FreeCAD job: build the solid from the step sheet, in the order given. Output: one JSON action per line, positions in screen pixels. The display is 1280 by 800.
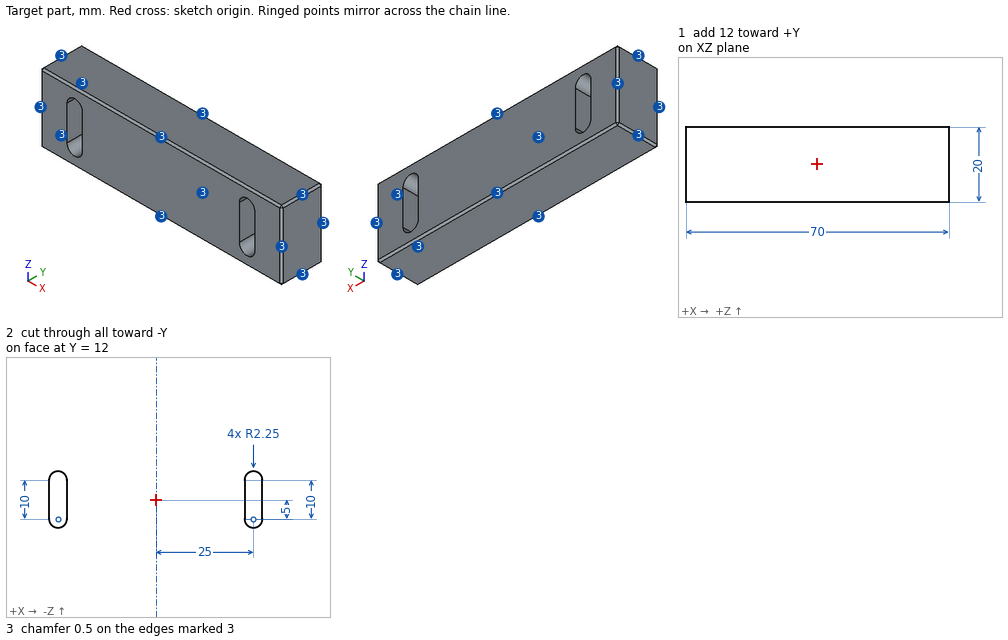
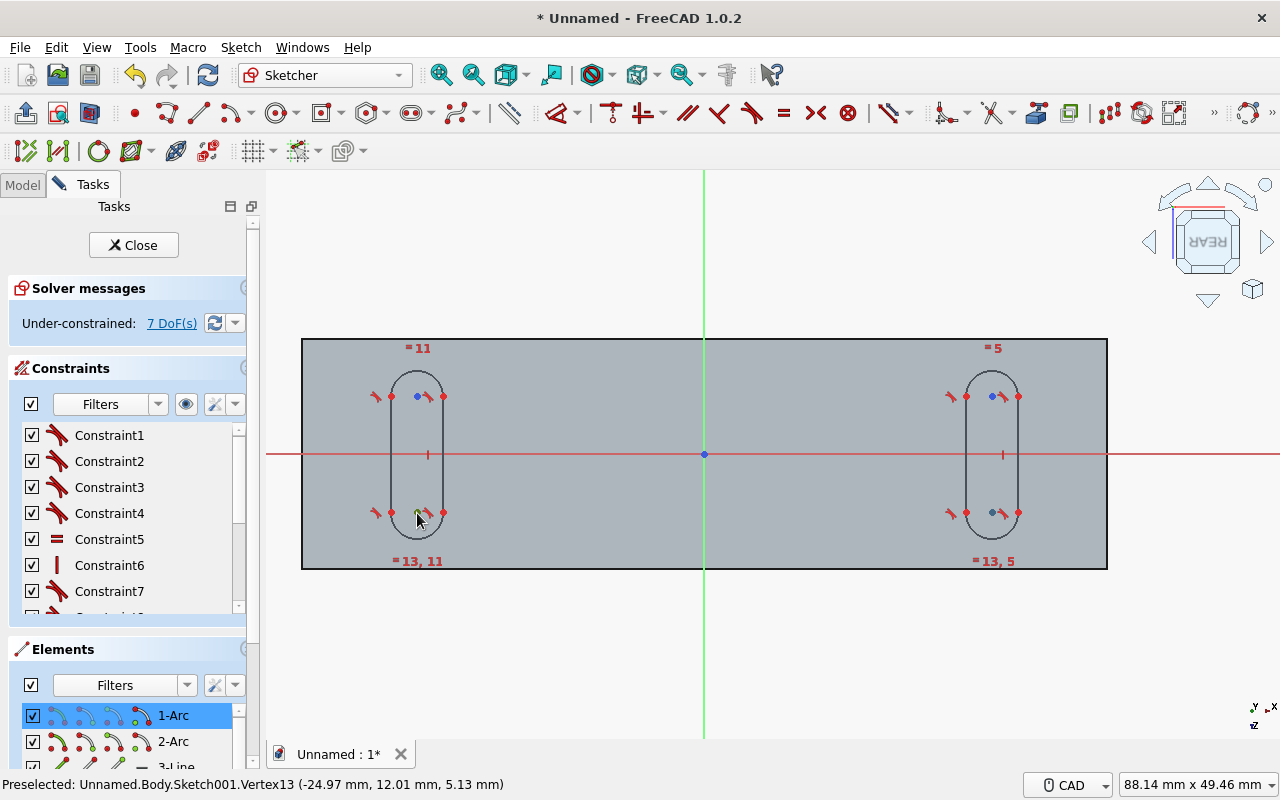
{"action": "left_click", "coordinate": [704, 674]}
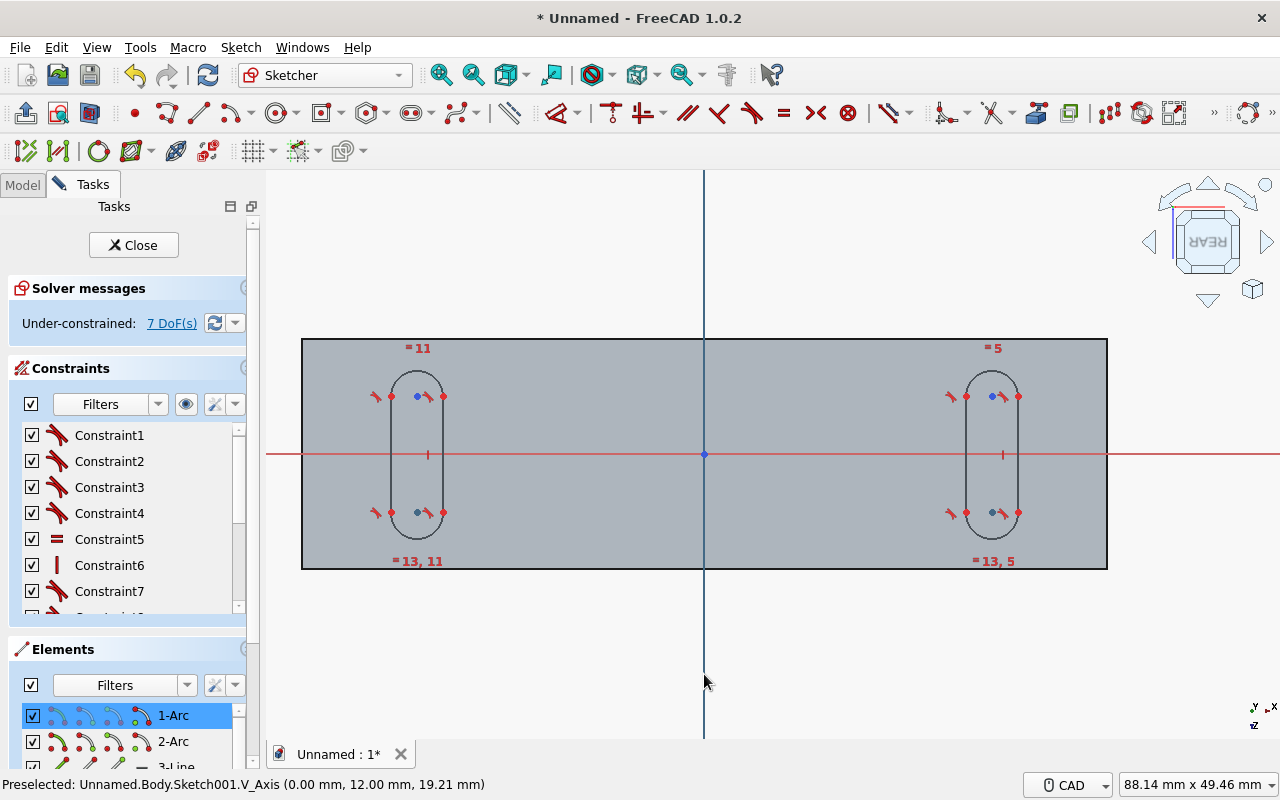
{"action": "key", "text": "s"}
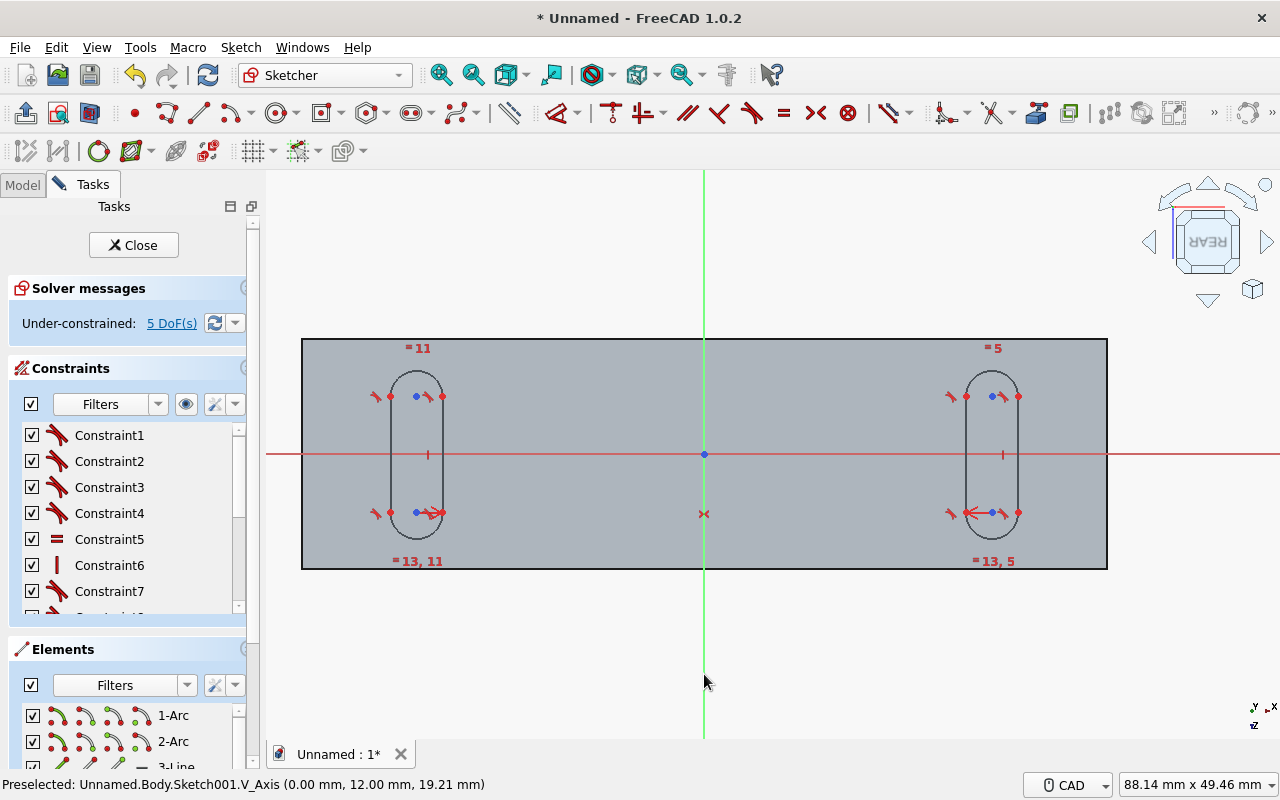
{"action": "scroll", "coordinate": [977, 534], "scroll_direction": "up", "scroll_amount": 3}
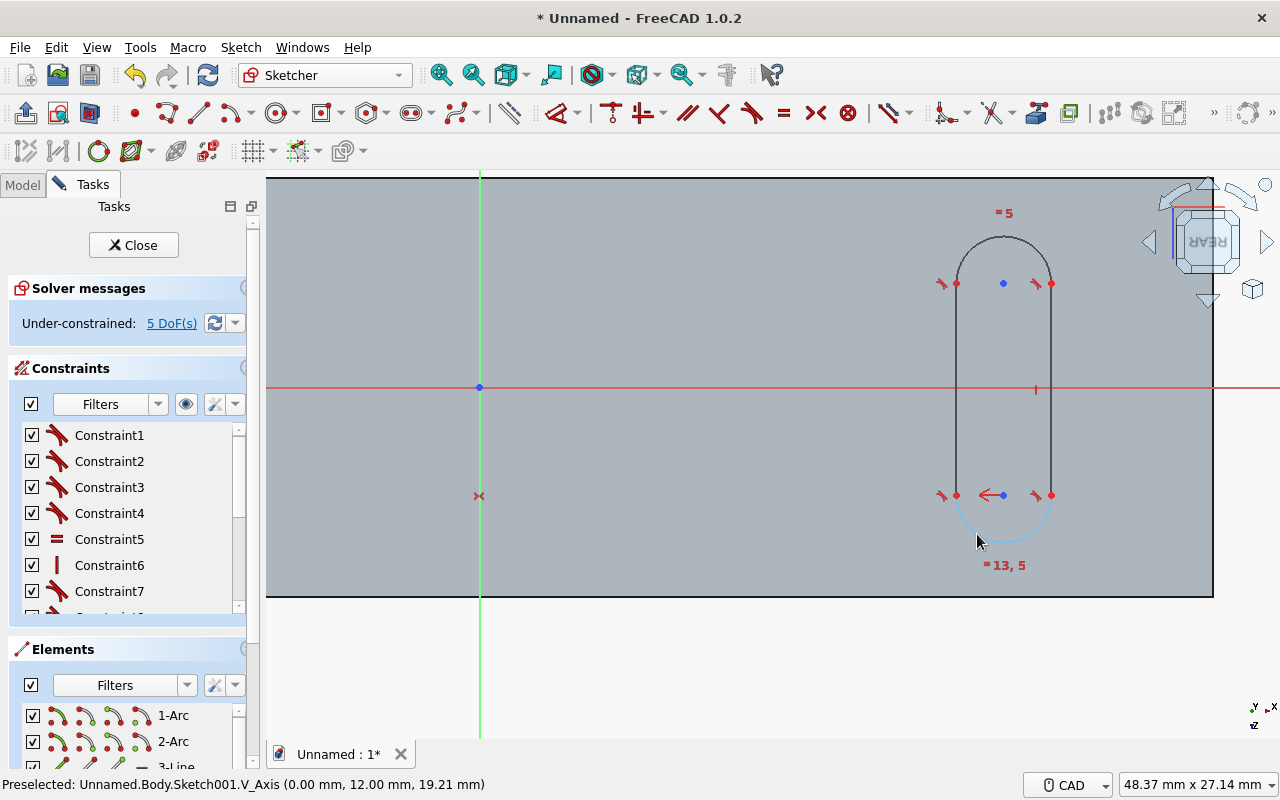
{"action": "left_click", "coordinate": [976, 534]}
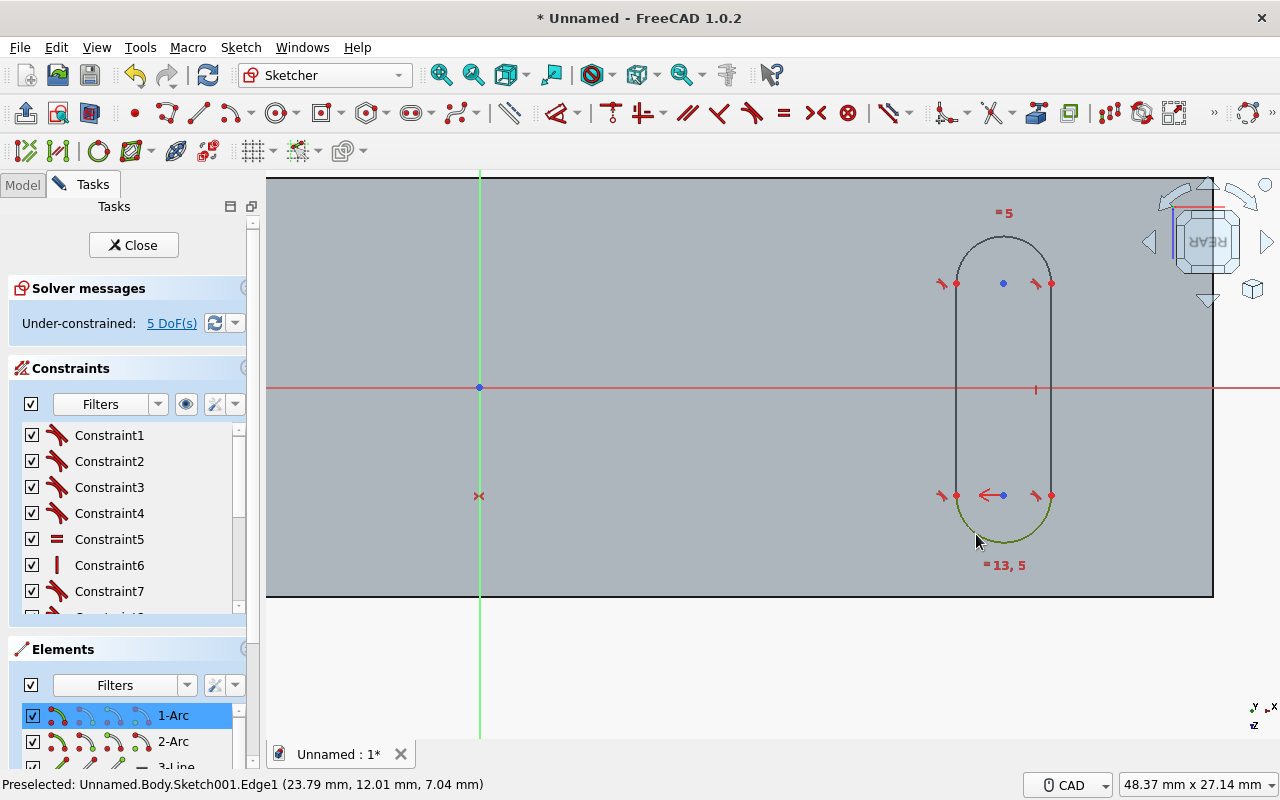
{"action": "left_click", "coordinate": [580, 114]}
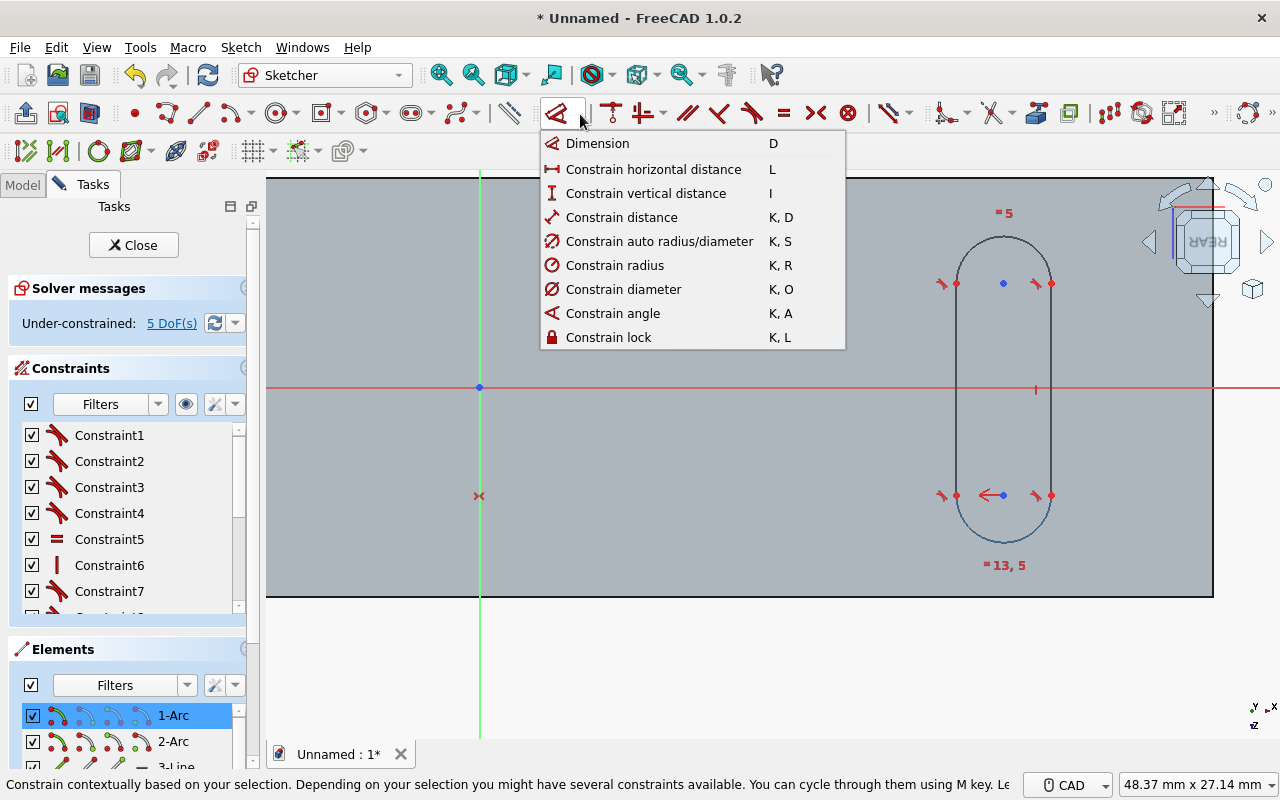
{"action": "left_click", "coordinate": [693, 265]}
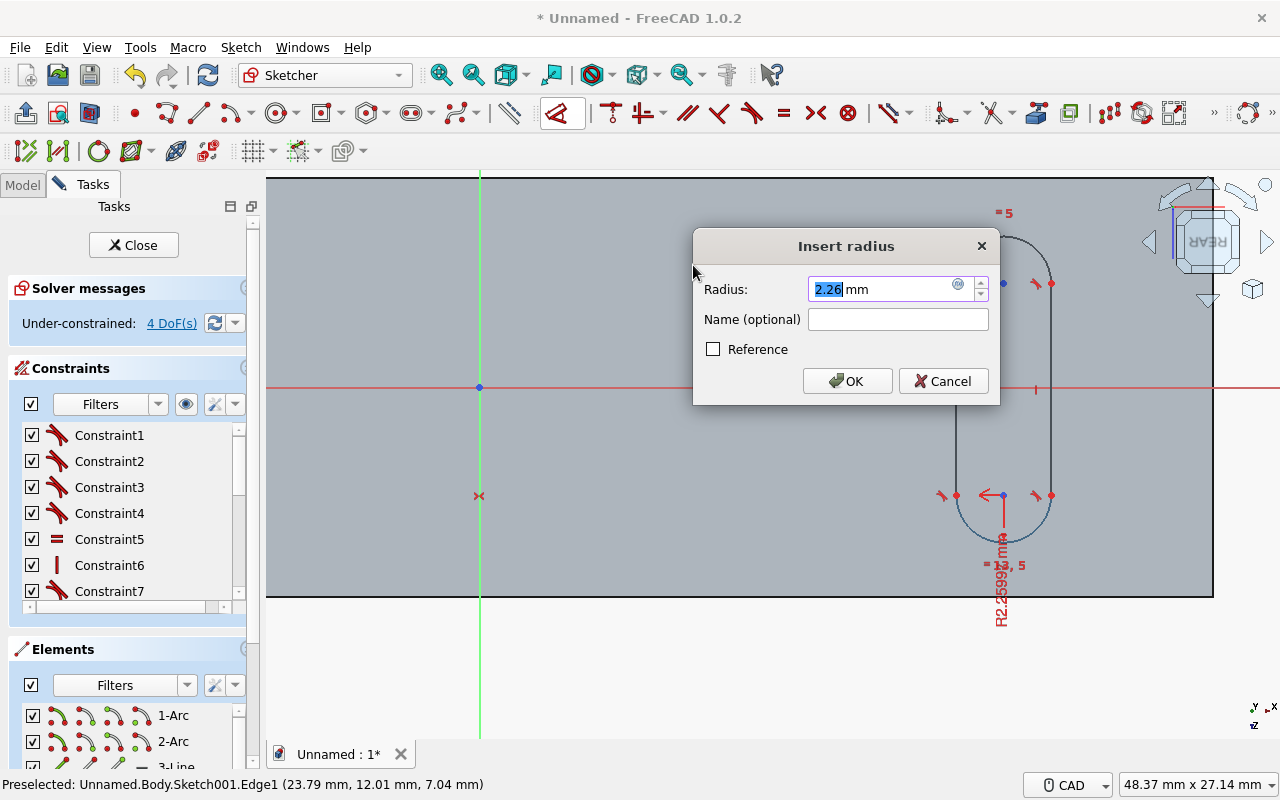
{"action": "type", "text": "2.25"}
{"action": "key", "text": "Return"}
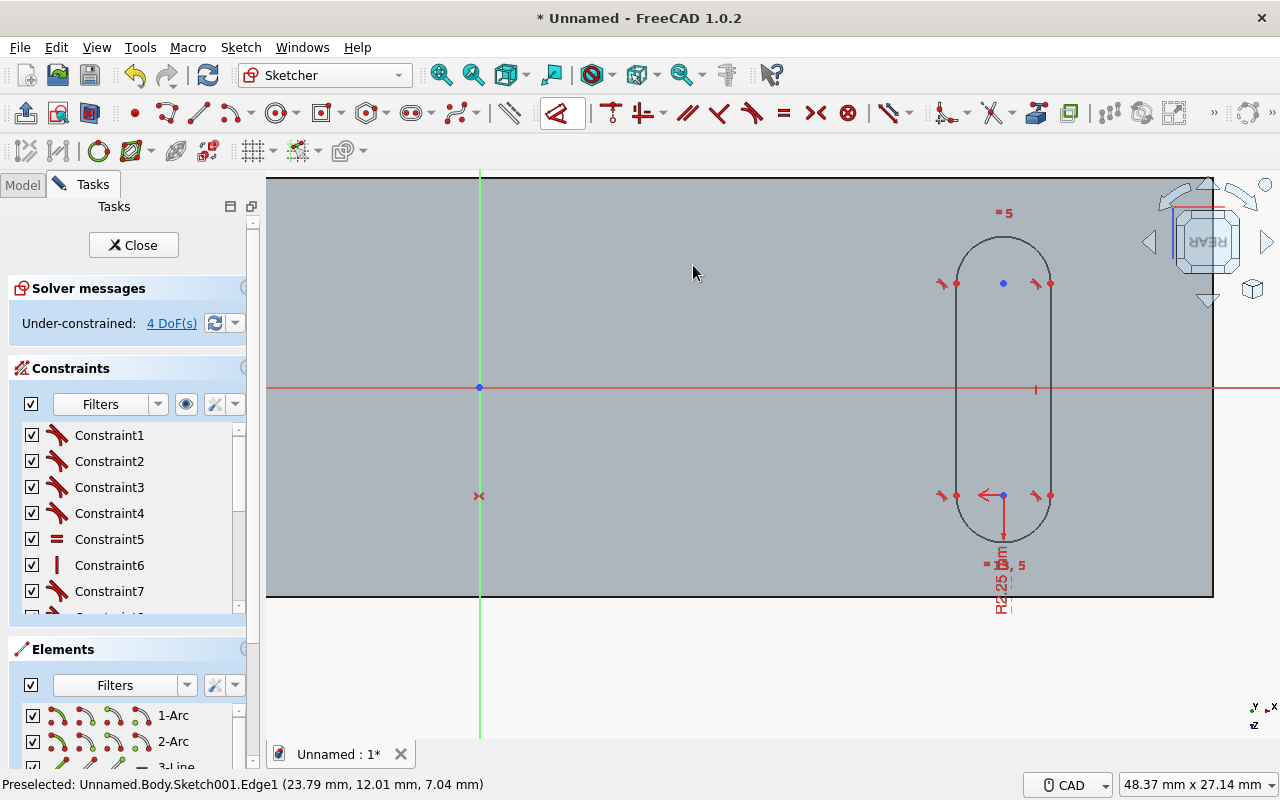
{"action": "left_click", "coordinate": [956, 432]}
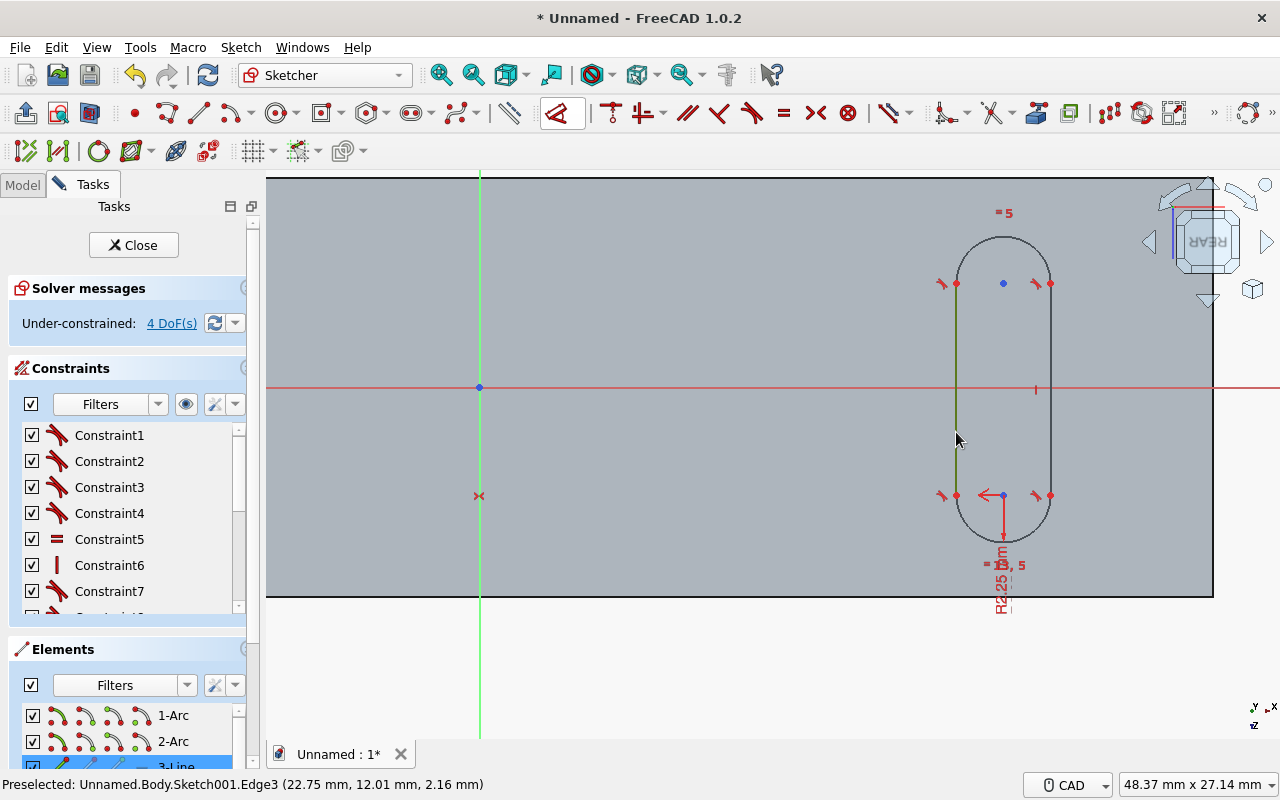
{"action": "left_click", "coordinate": [580, 114]}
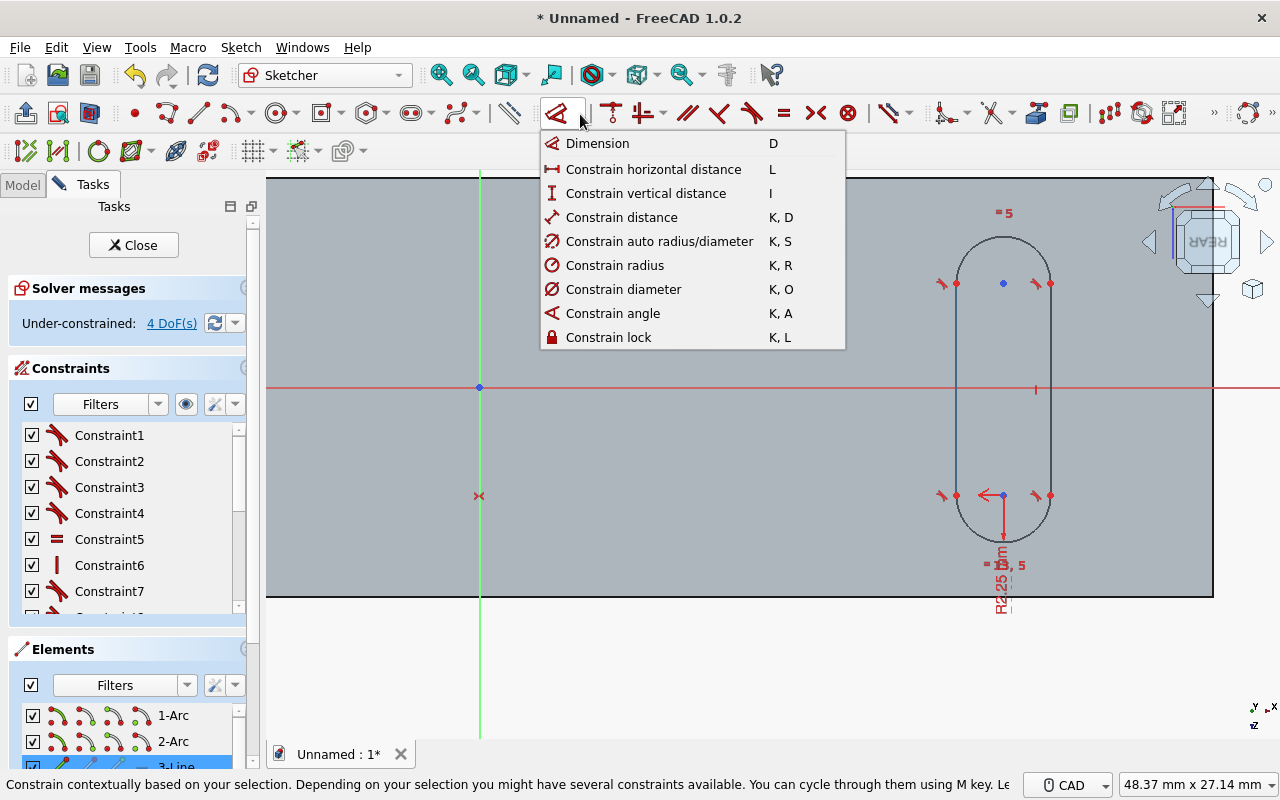
{"action": "left_click", "coordinate": [693, 193]}